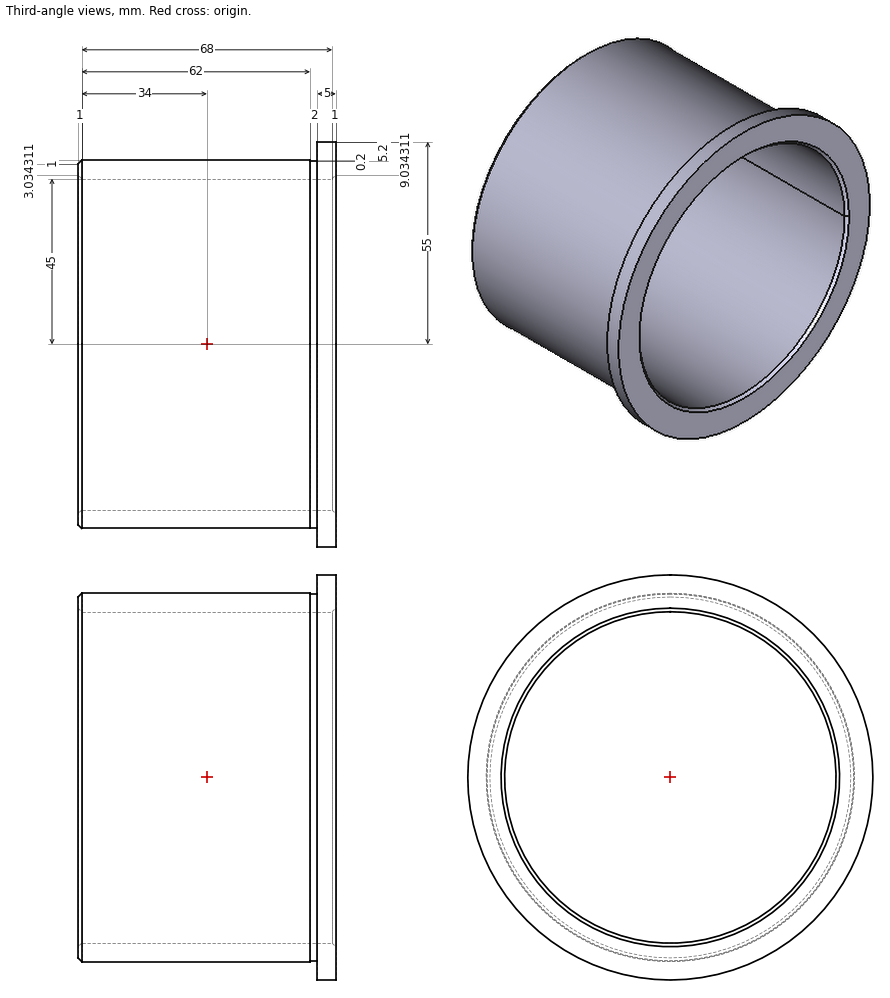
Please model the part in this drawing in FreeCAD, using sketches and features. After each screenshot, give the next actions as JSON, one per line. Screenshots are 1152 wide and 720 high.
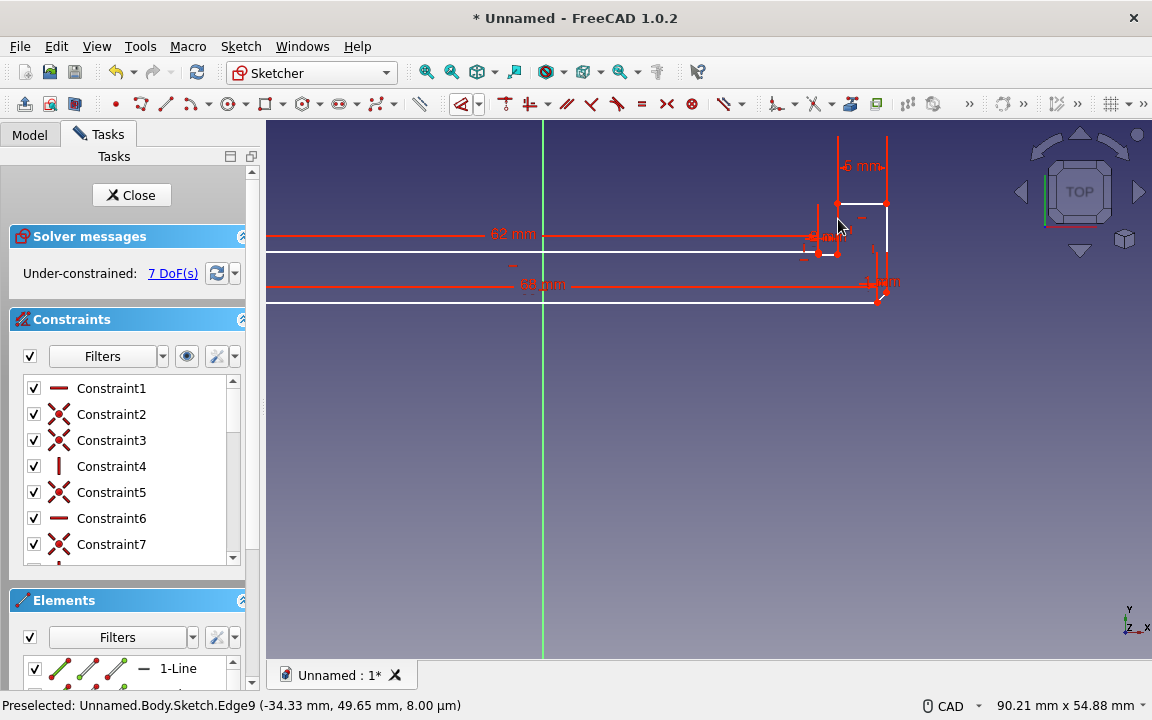
{"action": "left_click", "coordinate": [838, 219]}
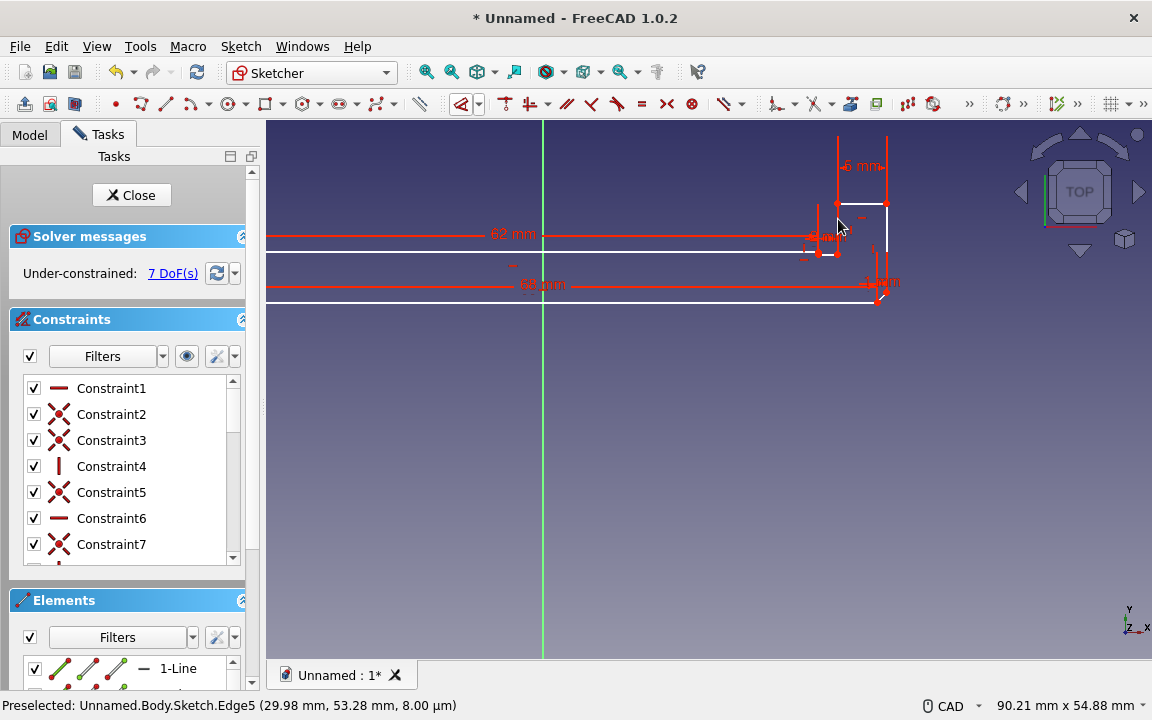
{"action": "key", "text": "i"}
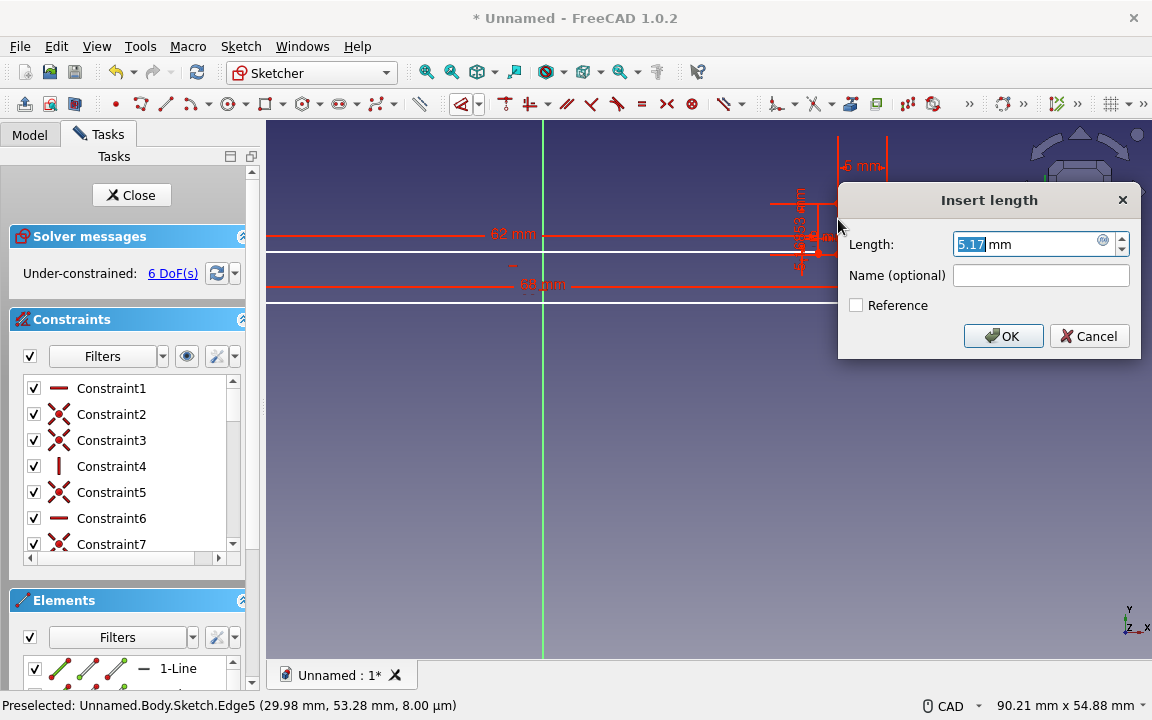
{"action": "type", "text": "5.2"}
{"action": "key", "text": "Return"}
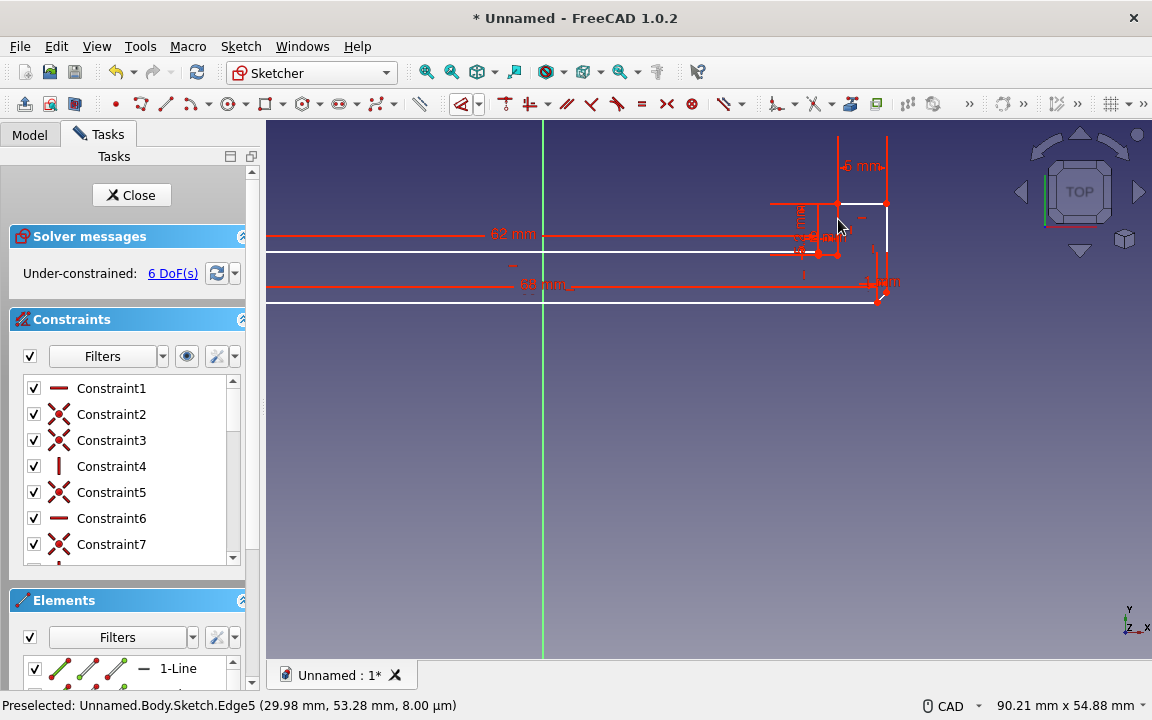
{"action": "scroll", "coordinate": [818, 254], "scroll_direction": "up", "scroll_amount": 16}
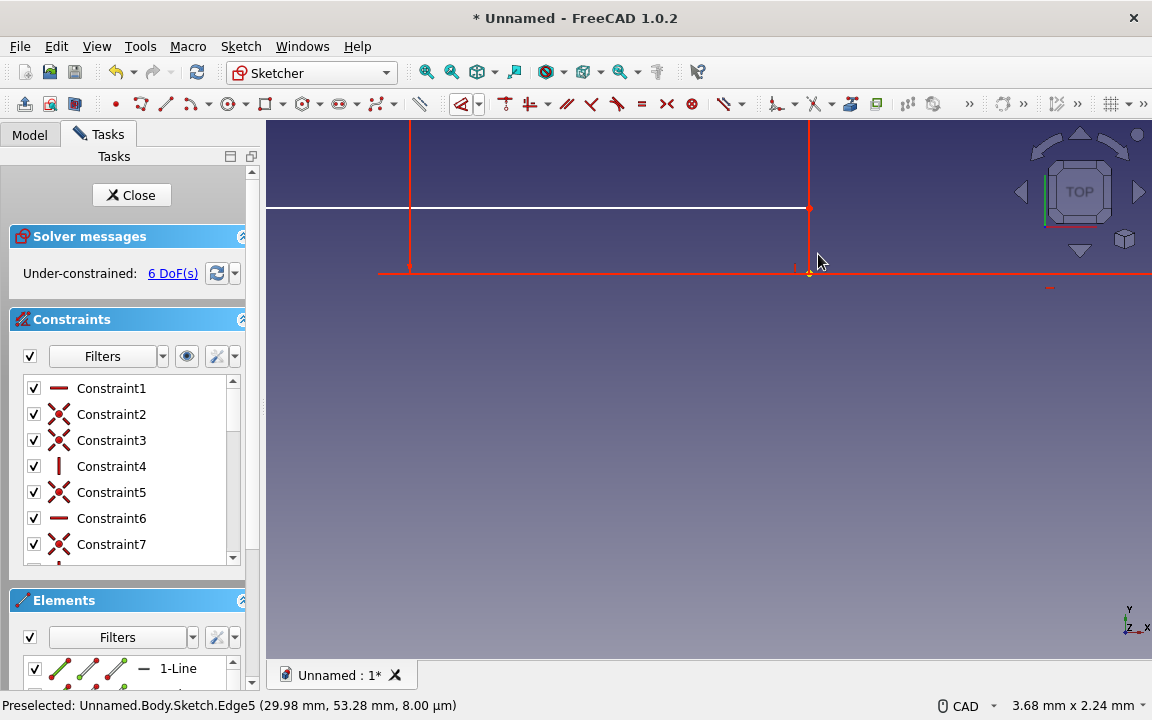
{"action": "left_click", "coordinate": [809, 241]}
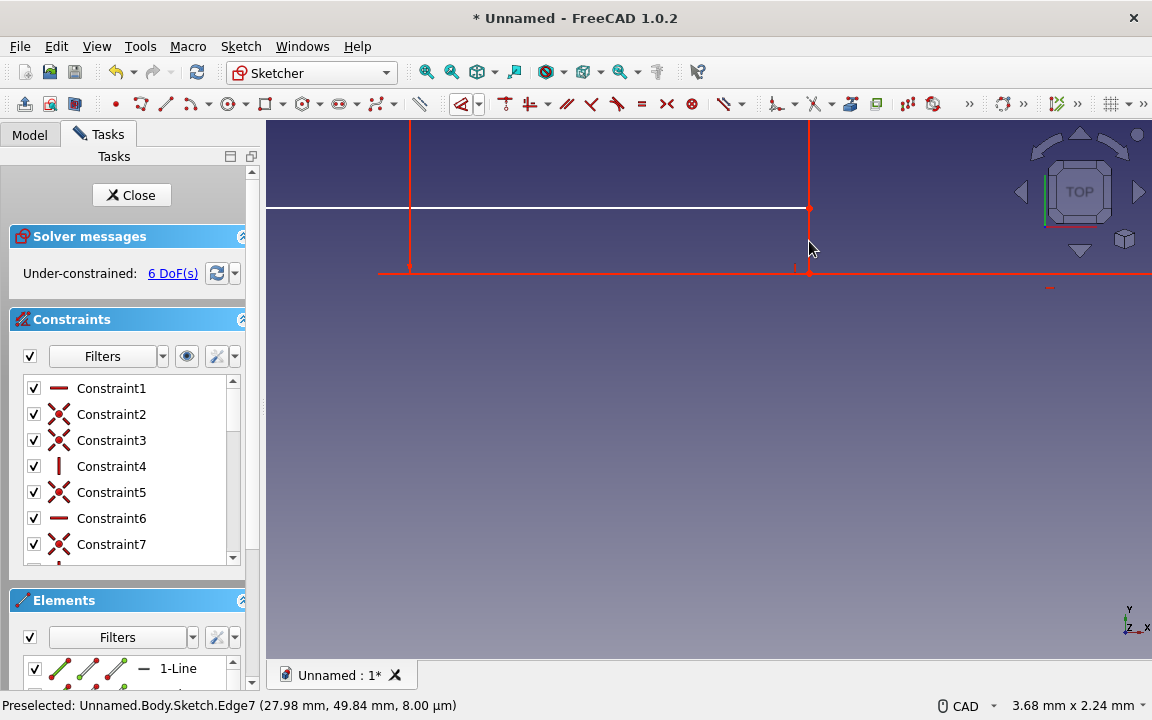
{"action": "key", "text": "i"}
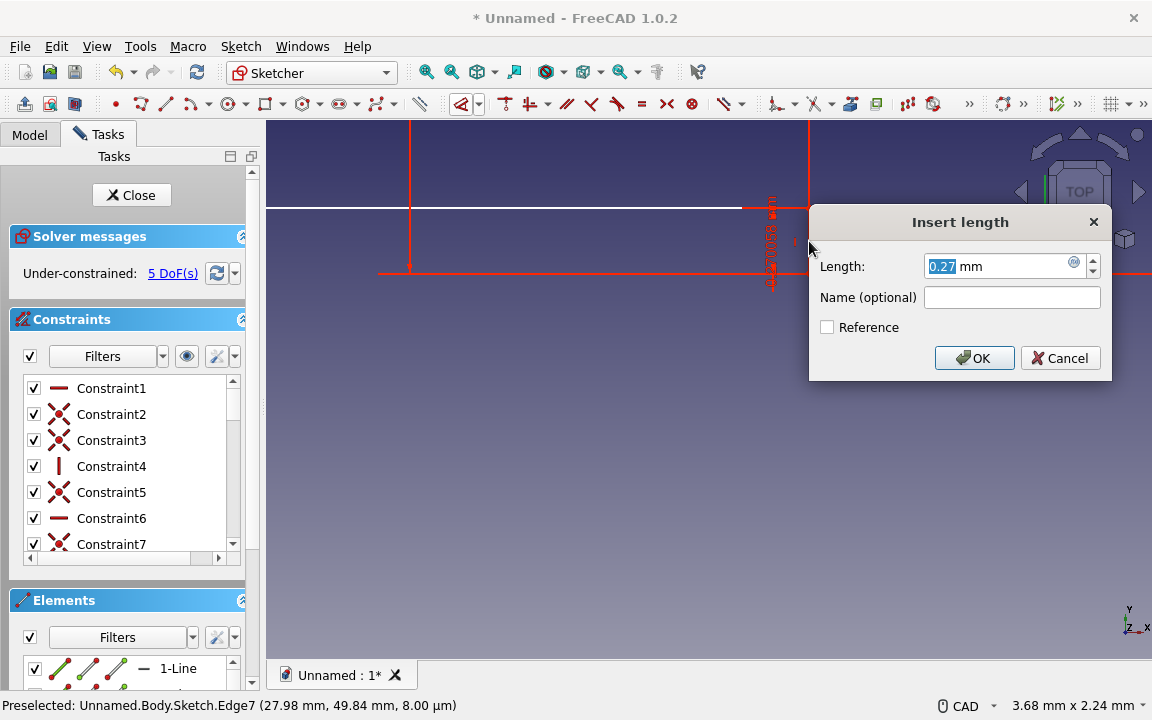
{"action": "type", "text": "0.2"}
{"action": "key", "text": "Return"}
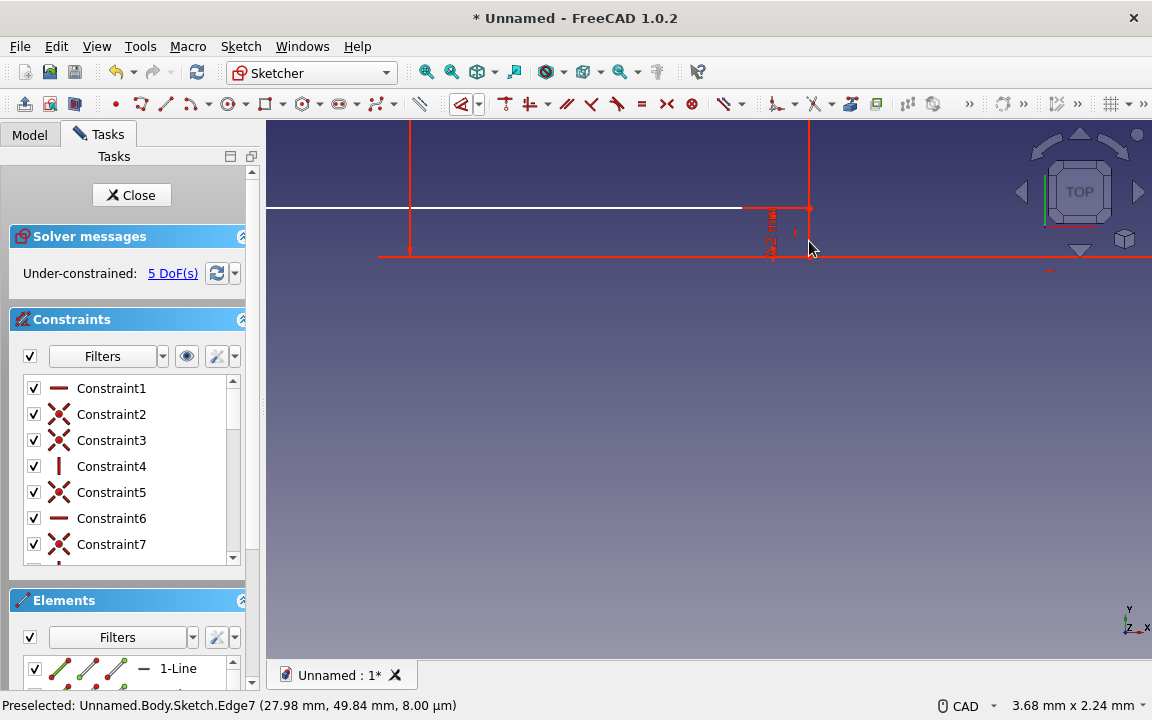
{"action": "scroll", "coordinate": [825, 242], "scroll_direction": "down", "scroll_amount": 18}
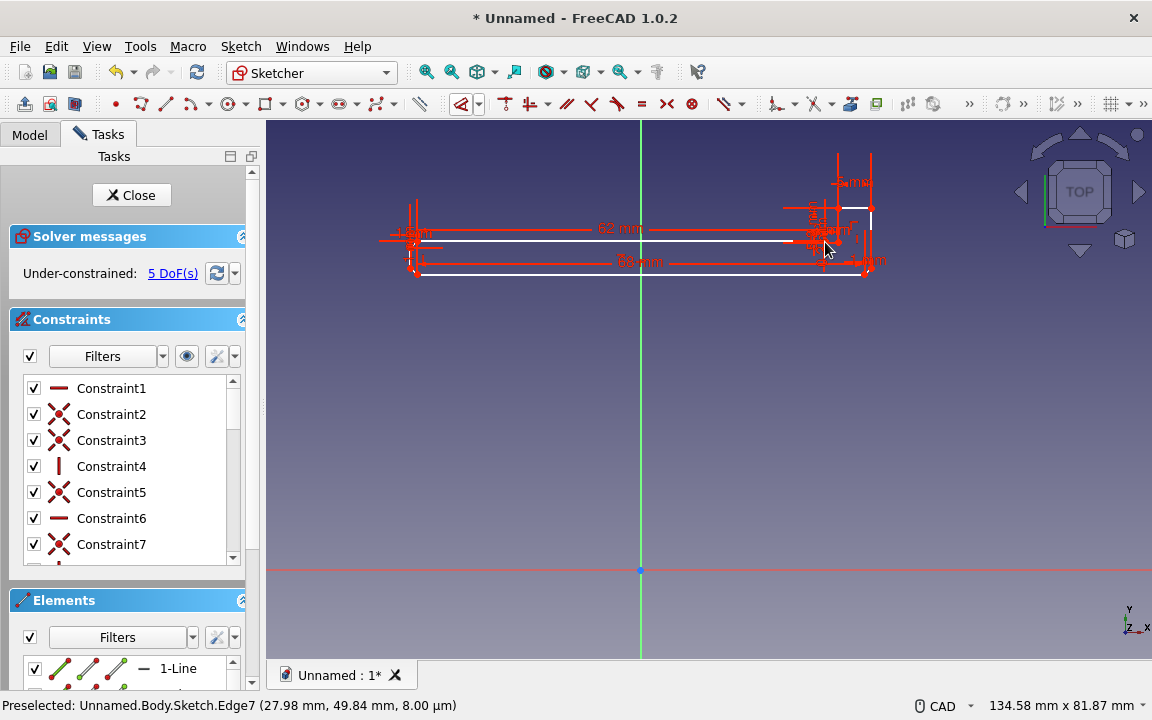
{"action": "scroll", "coordinate": [417, 275], "scroll_direction": "up", "scroll_amount": 2}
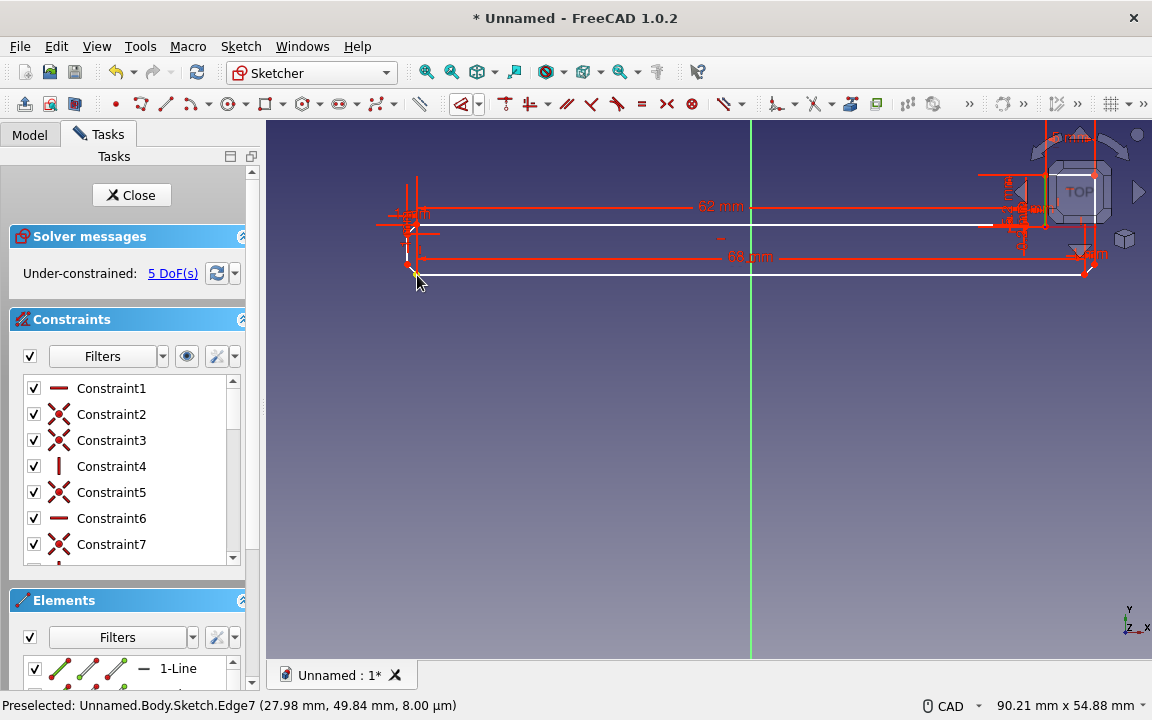
{"action": "left_click", "coordinate": [417, 275]}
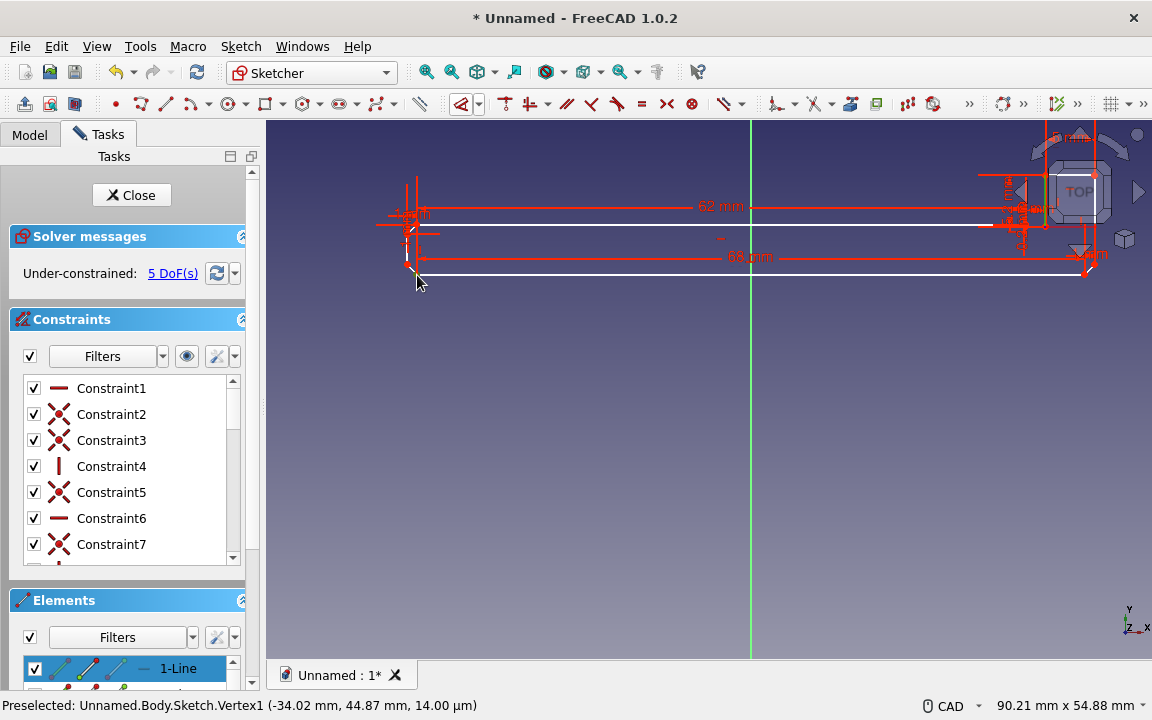
{"action": "key", "text": "l"}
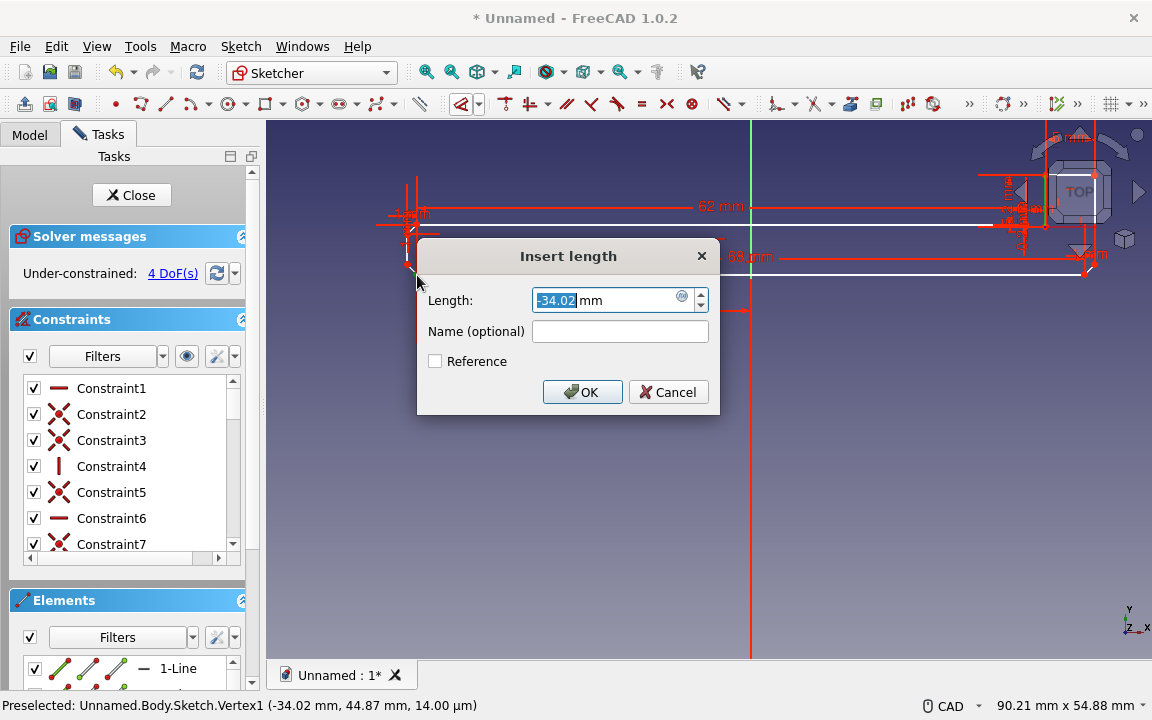
{"action": "type", "text": "-34"}
{"action": "key", "text": "Return"}